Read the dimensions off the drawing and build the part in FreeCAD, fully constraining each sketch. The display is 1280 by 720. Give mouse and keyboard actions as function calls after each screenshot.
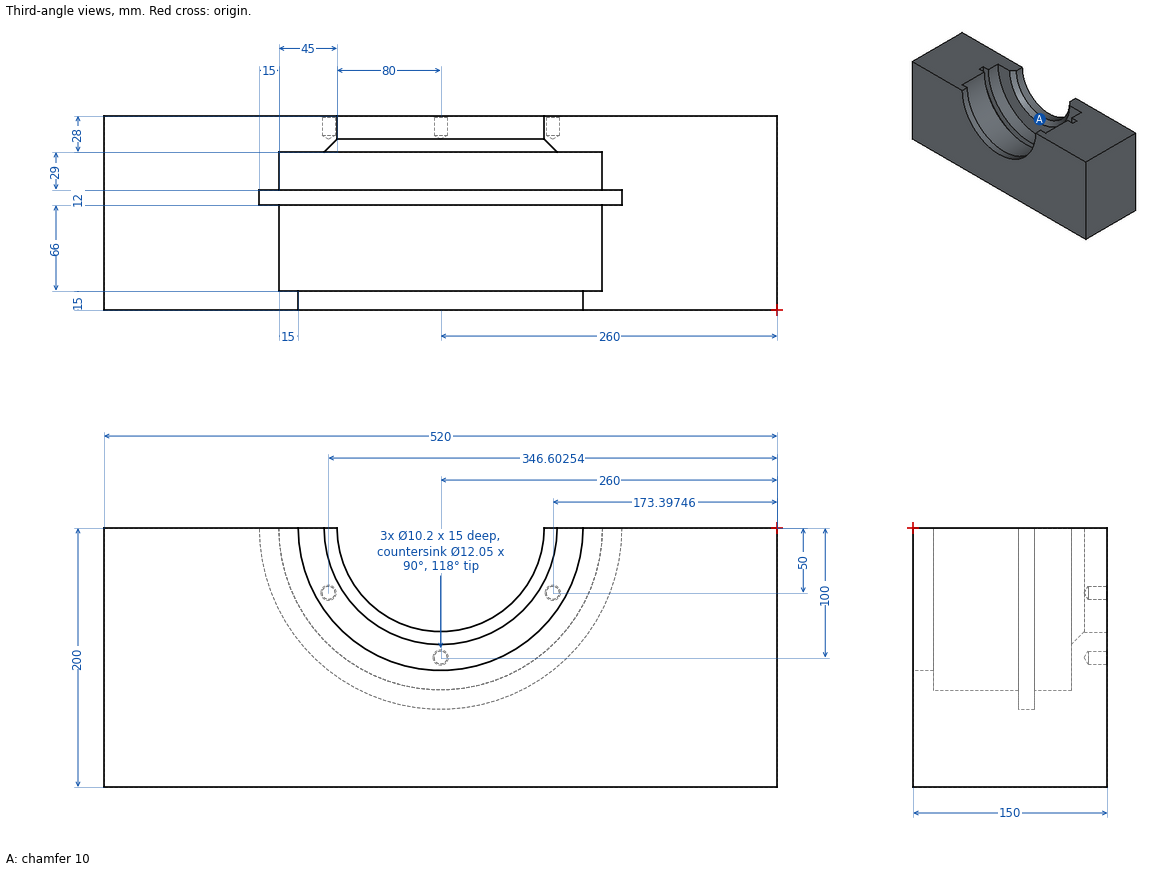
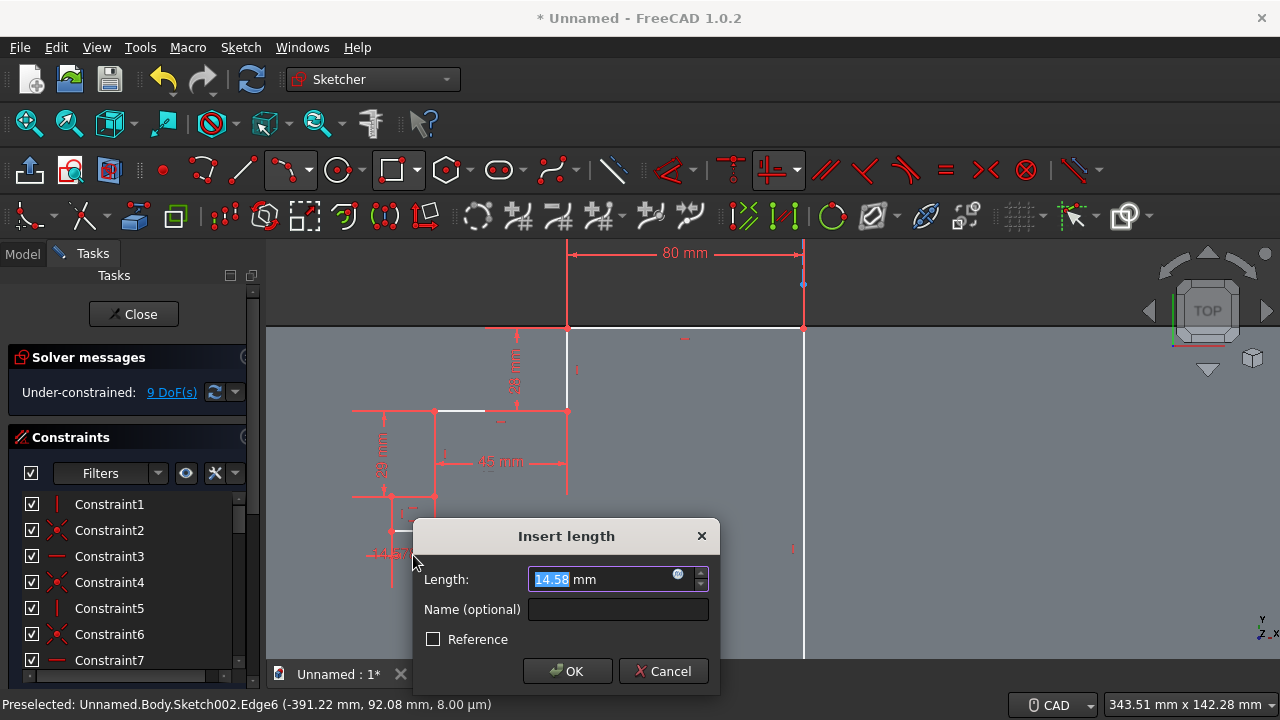
text(15)
key(Return)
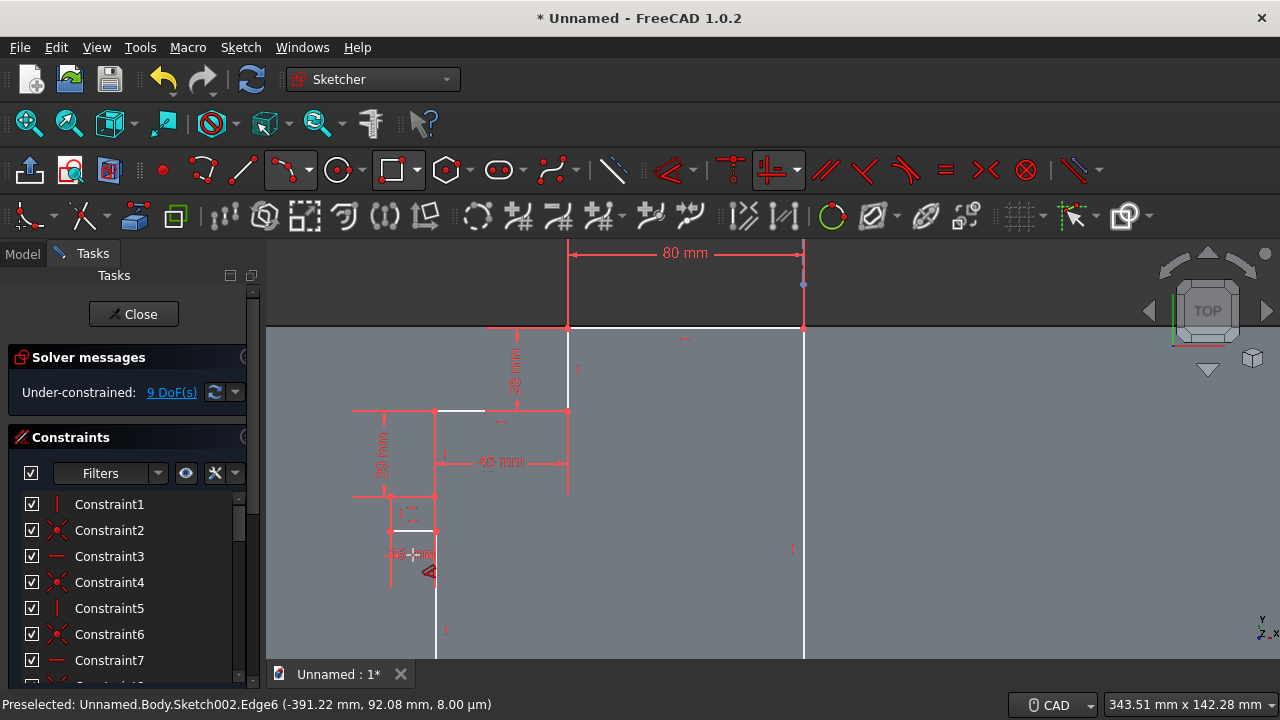
scroll(391, 507, up, 2)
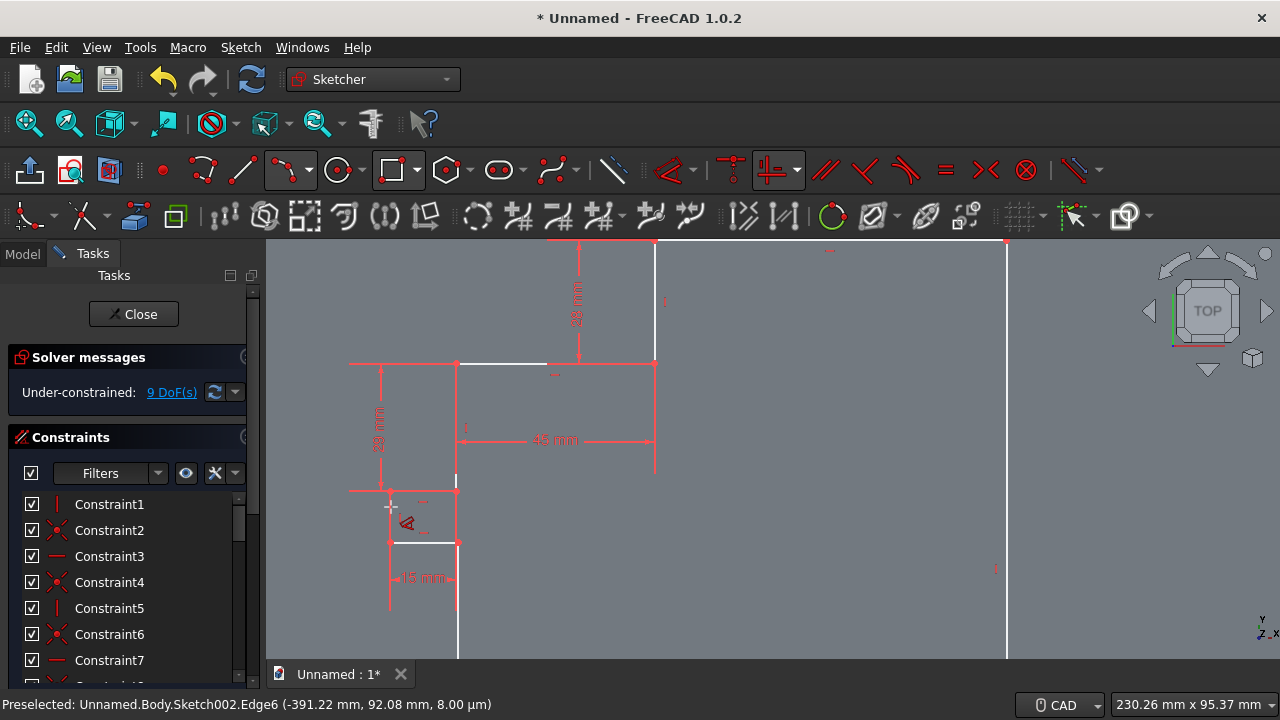
click(390, 507)
click(356, 517)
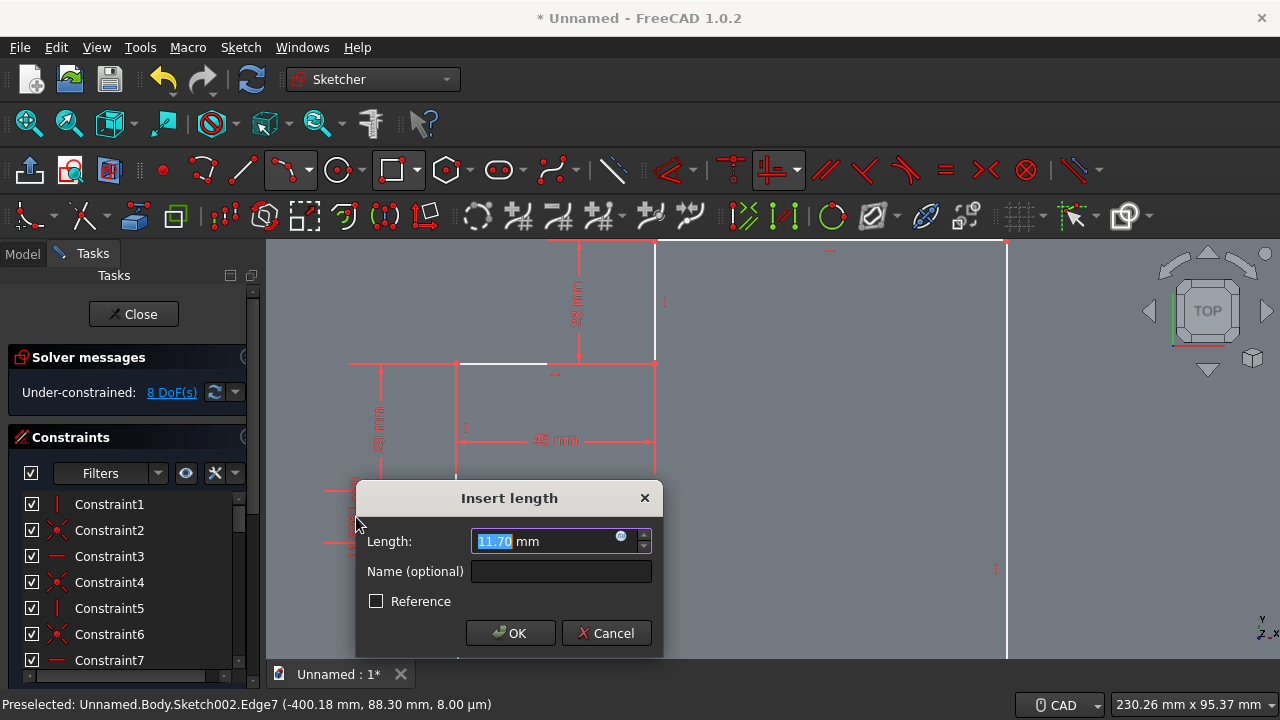
text(12)
key(Return)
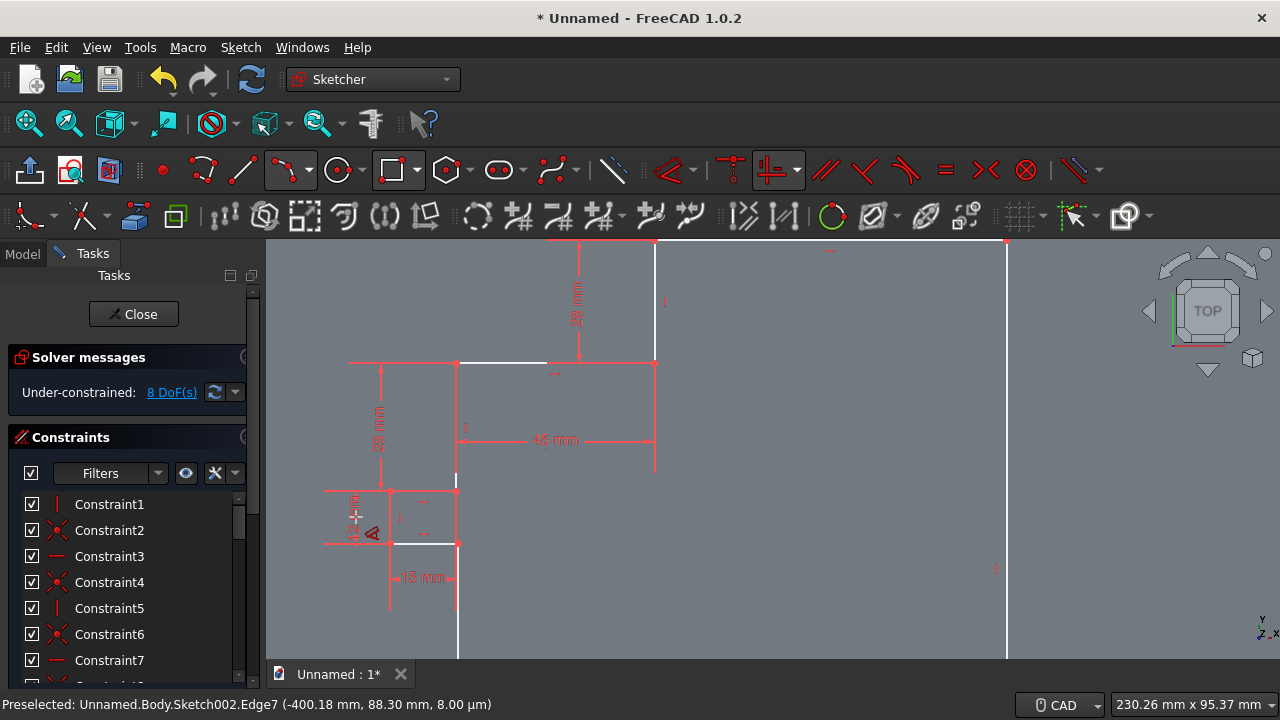
click(411, 544)
click(440, 510)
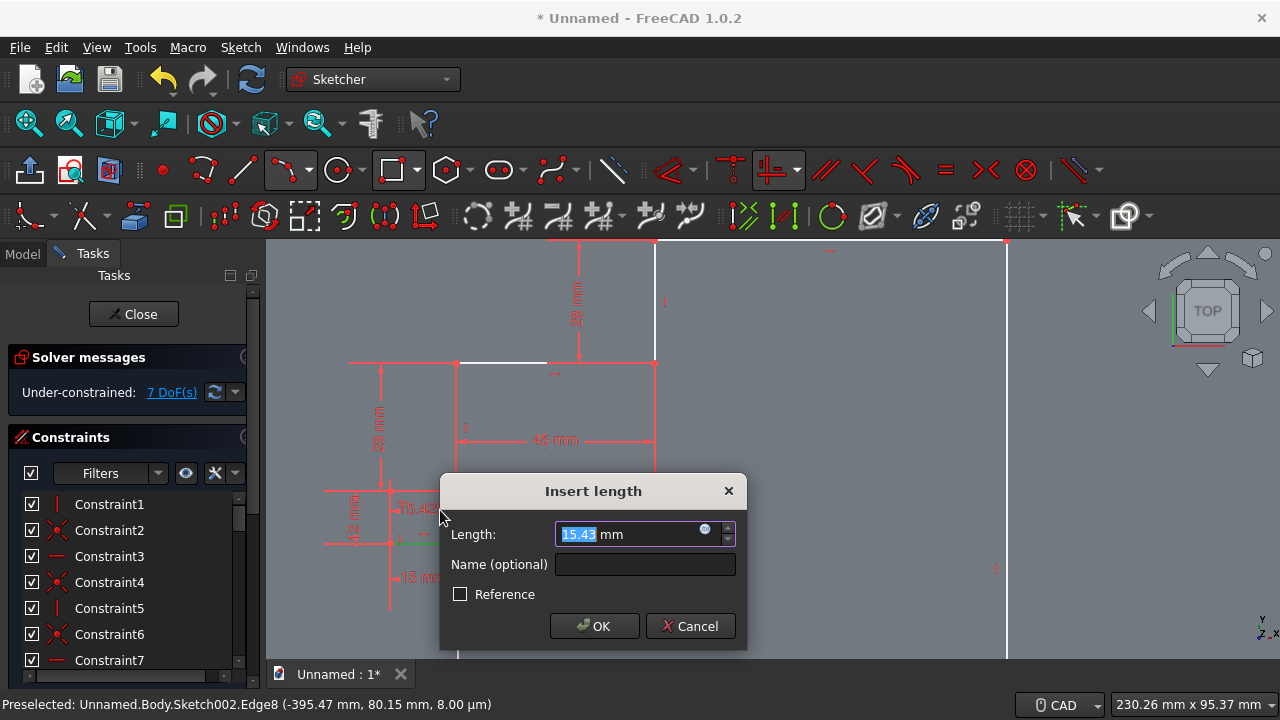
text(15)
key(Return)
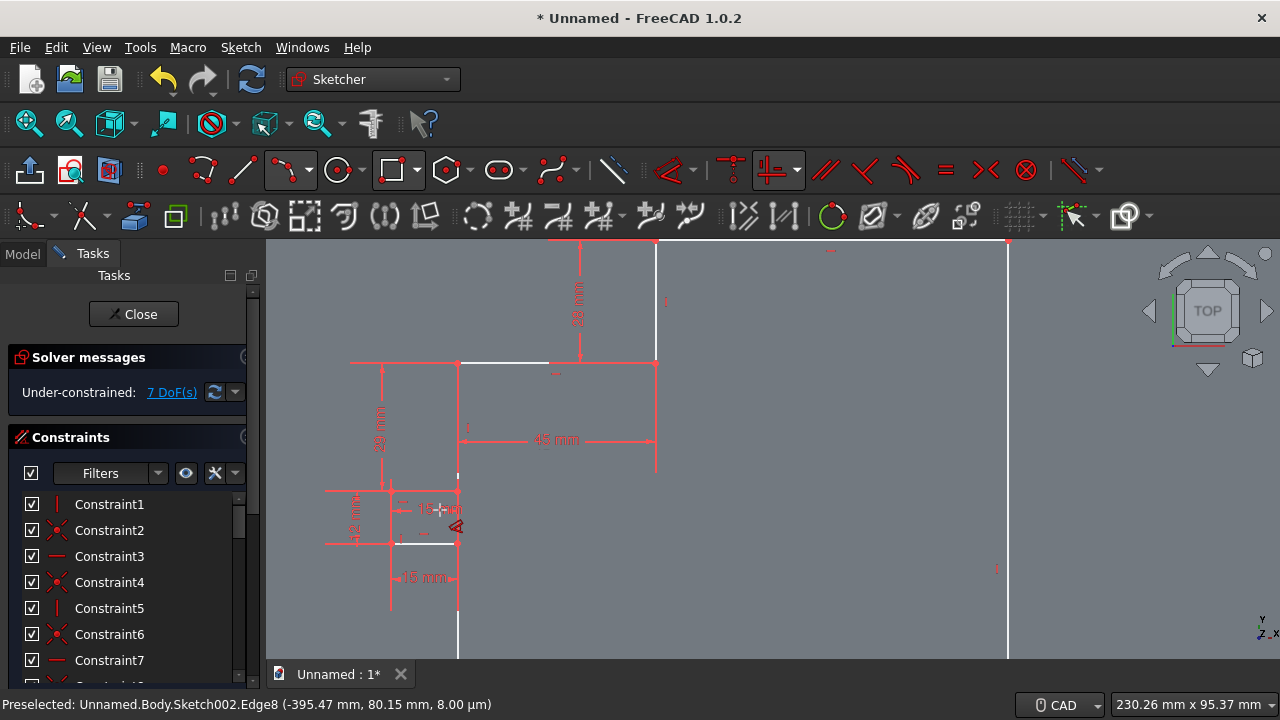
click(458, 602)
click(424, 607)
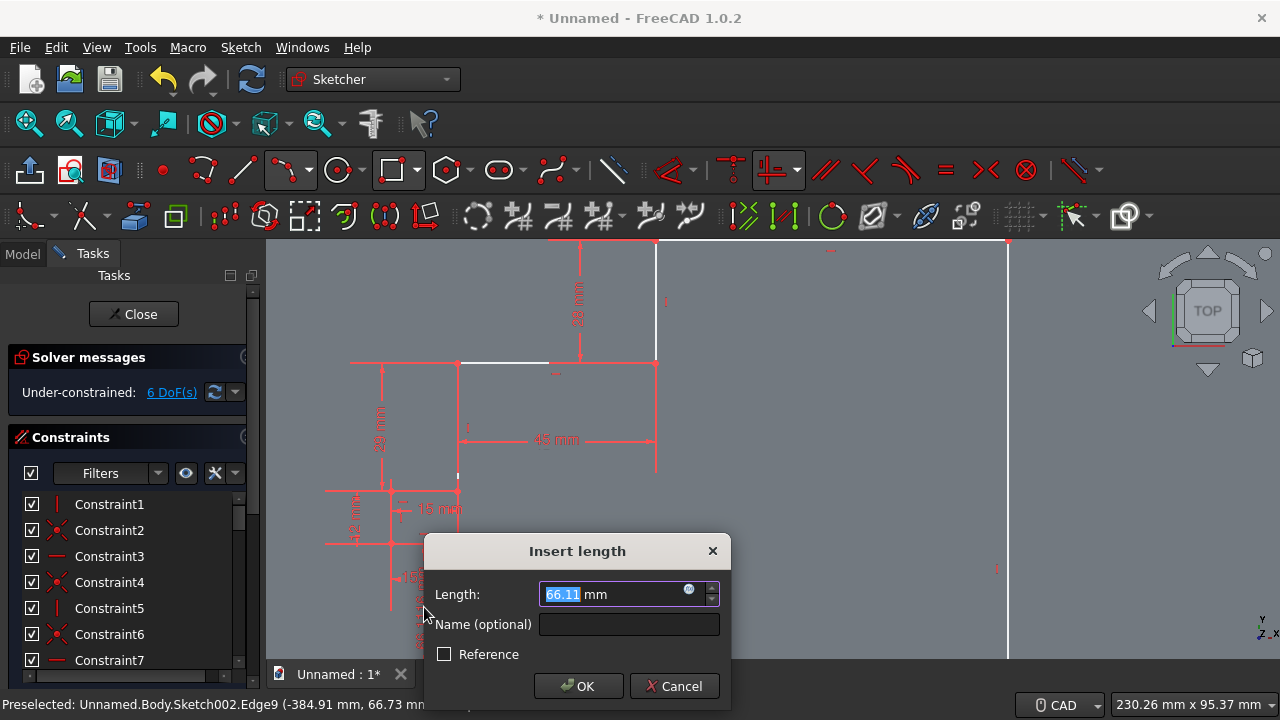
text(66)
key(Return)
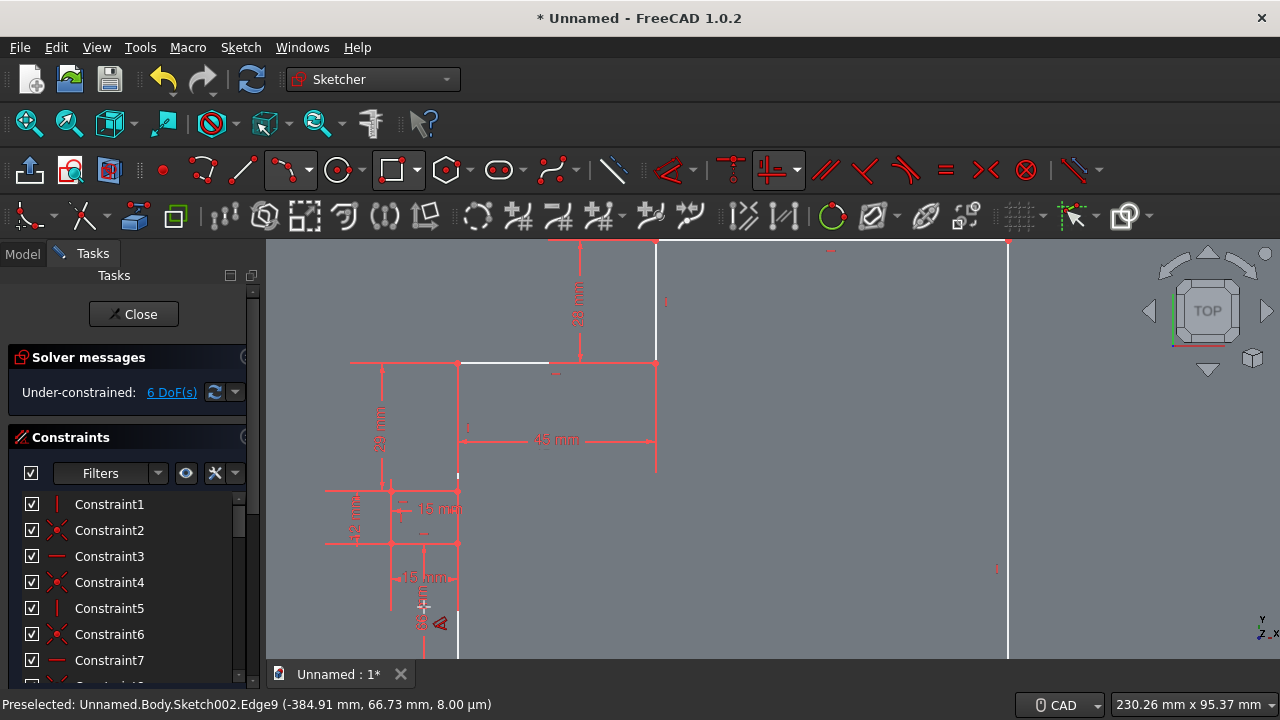
scroll(460, 455, down, 6)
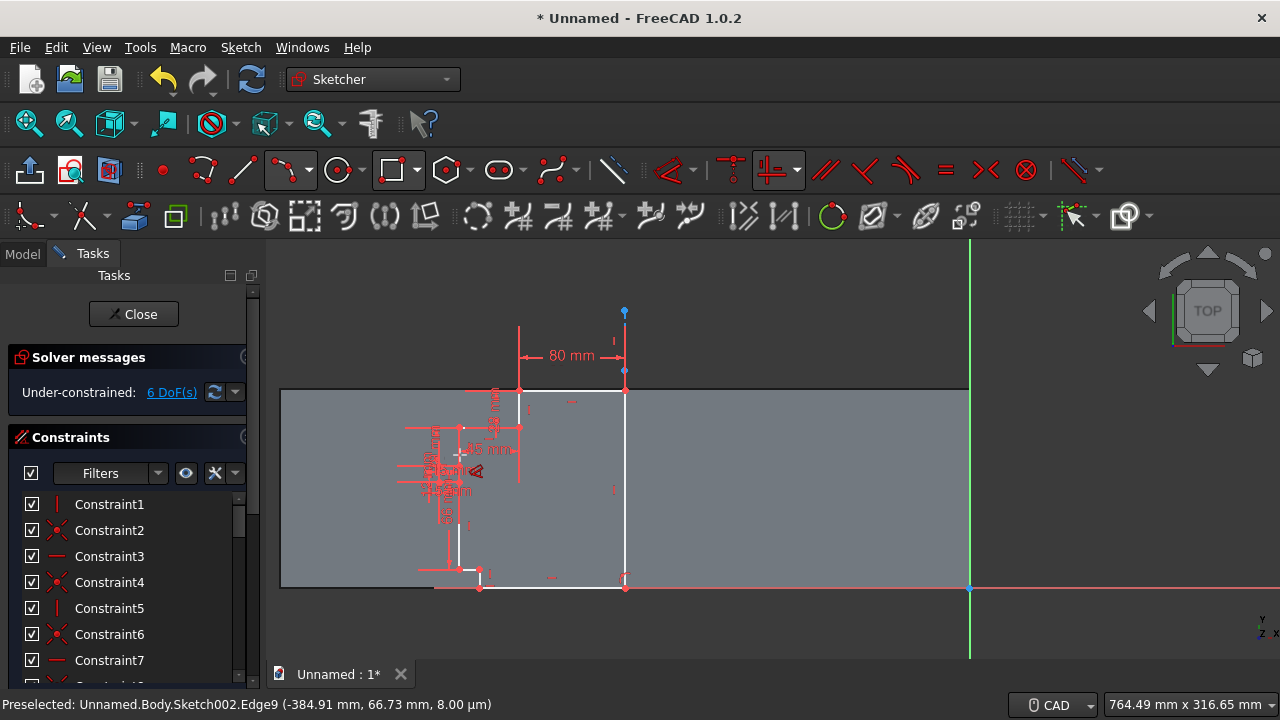
scroll(465, 570, up, 5)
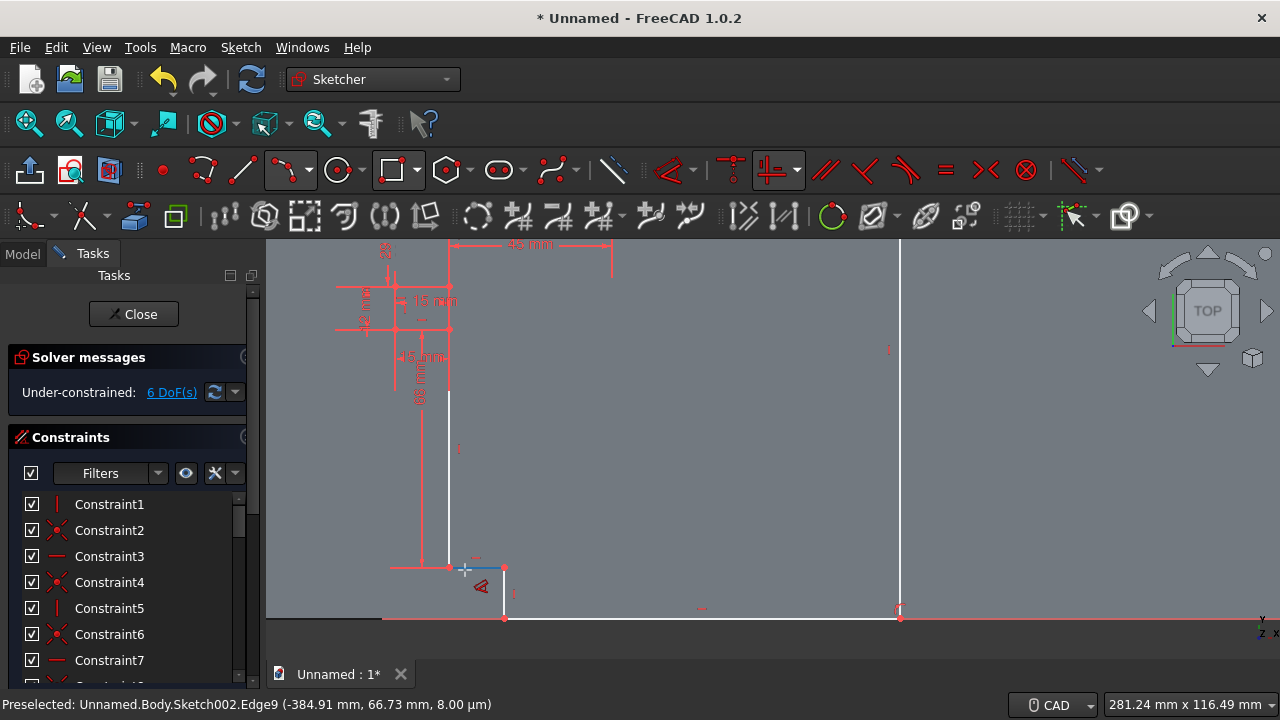
click(466, 568)
click(477, 602)